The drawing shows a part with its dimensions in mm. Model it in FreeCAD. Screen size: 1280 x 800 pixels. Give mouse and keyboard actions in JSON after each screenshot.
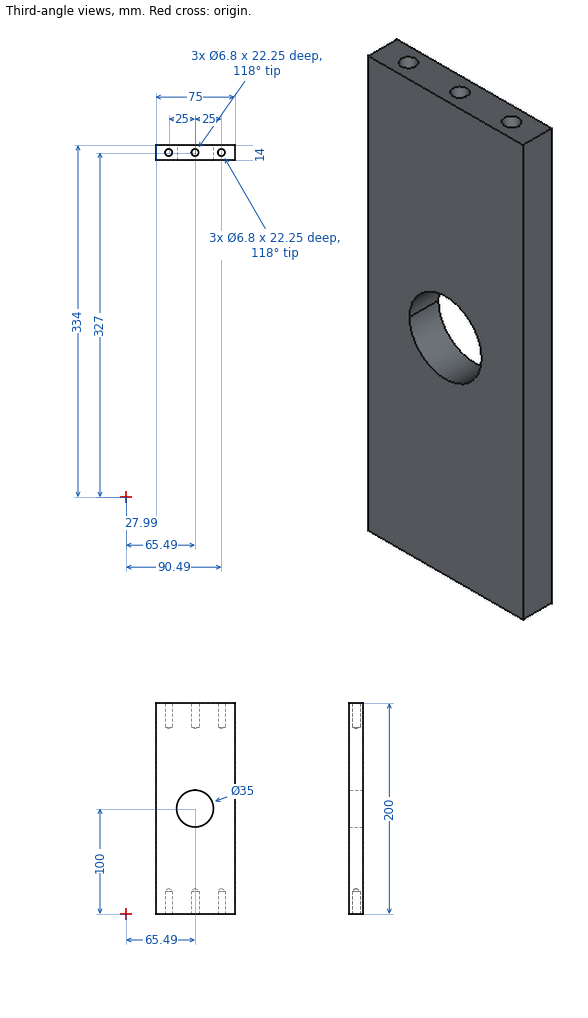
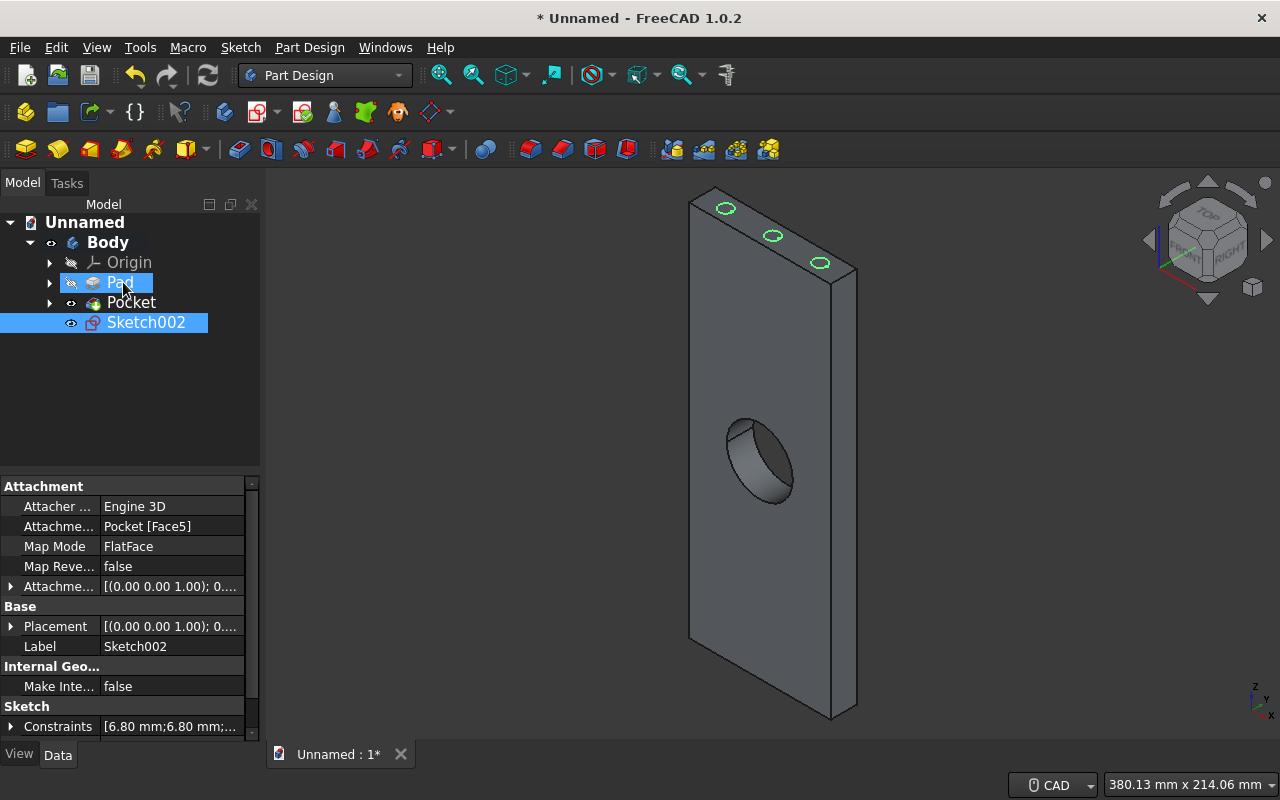
{"action": "left_click", "coordinate": [272, 150]}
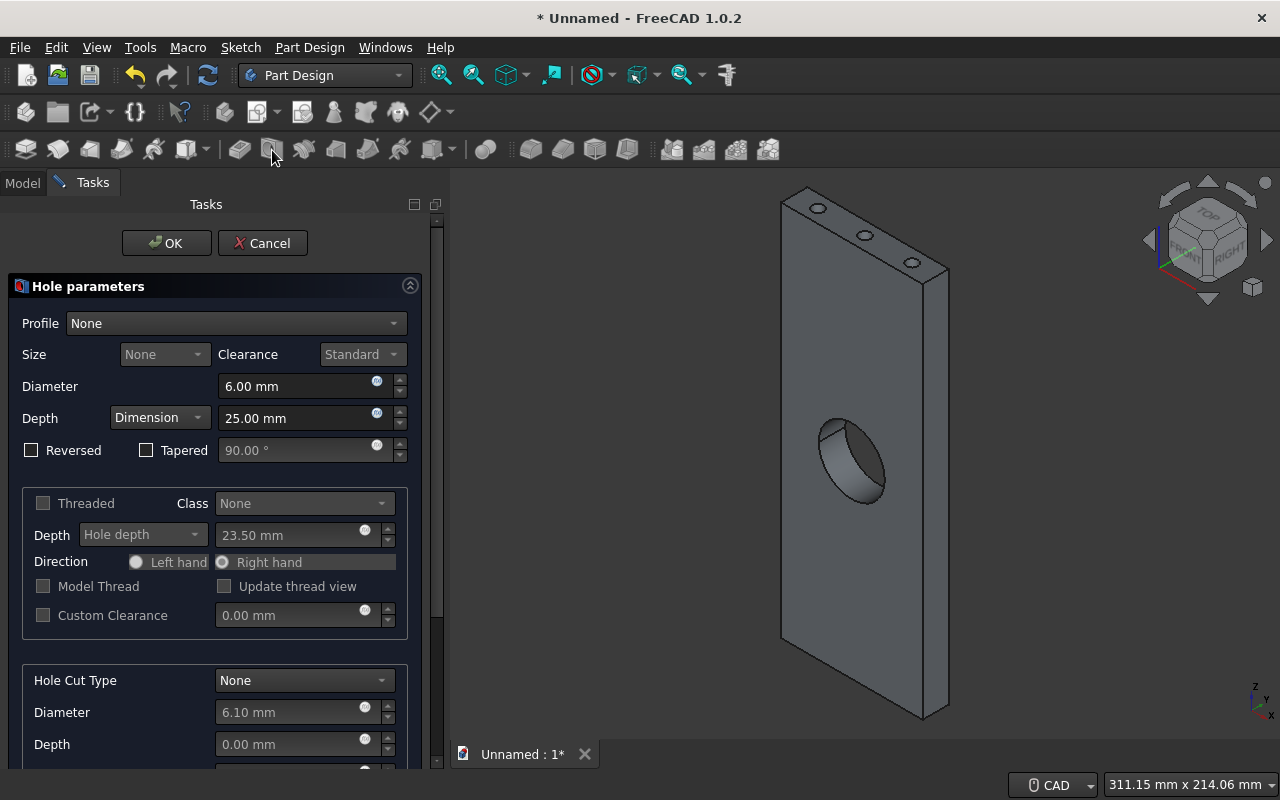
{"action": "triple_click", "coordinate": [305, 386]}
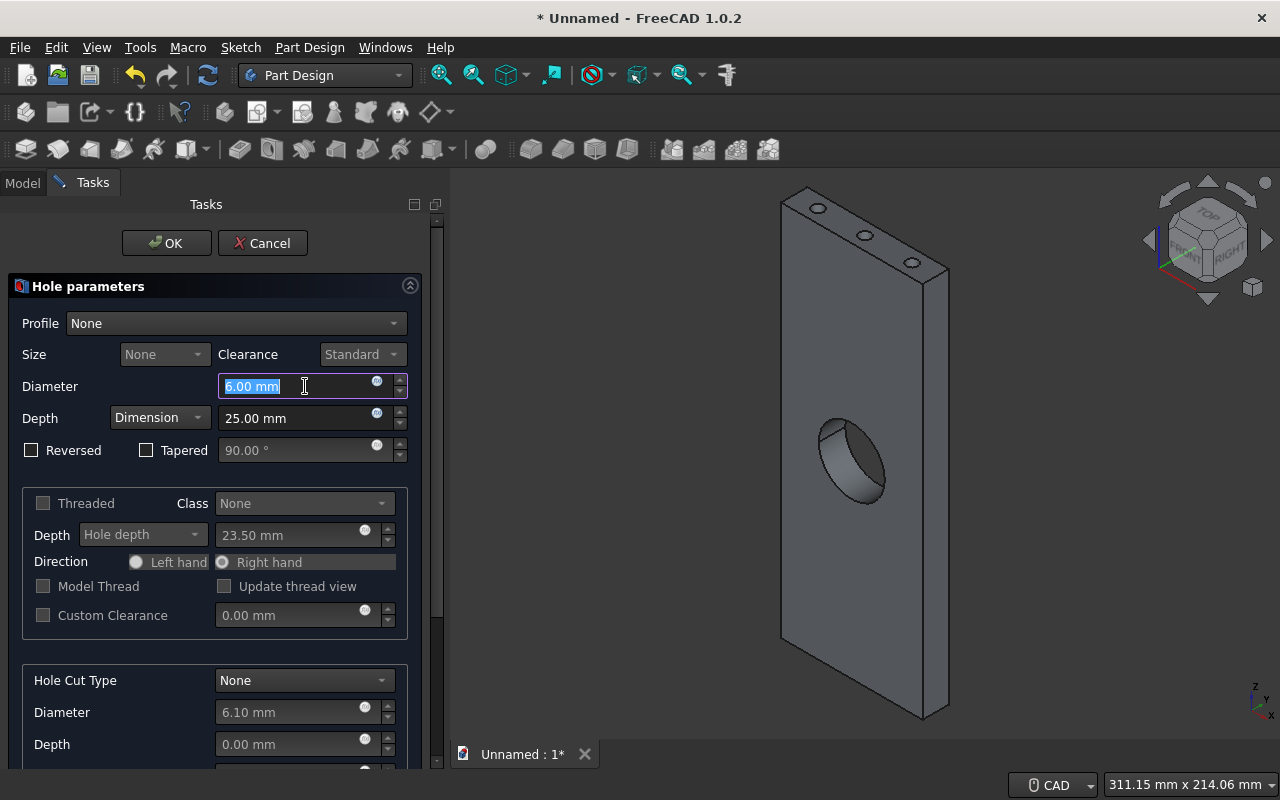
{"action": "type", "text": "6.8"}
{"action": "key", "text": "Tab"}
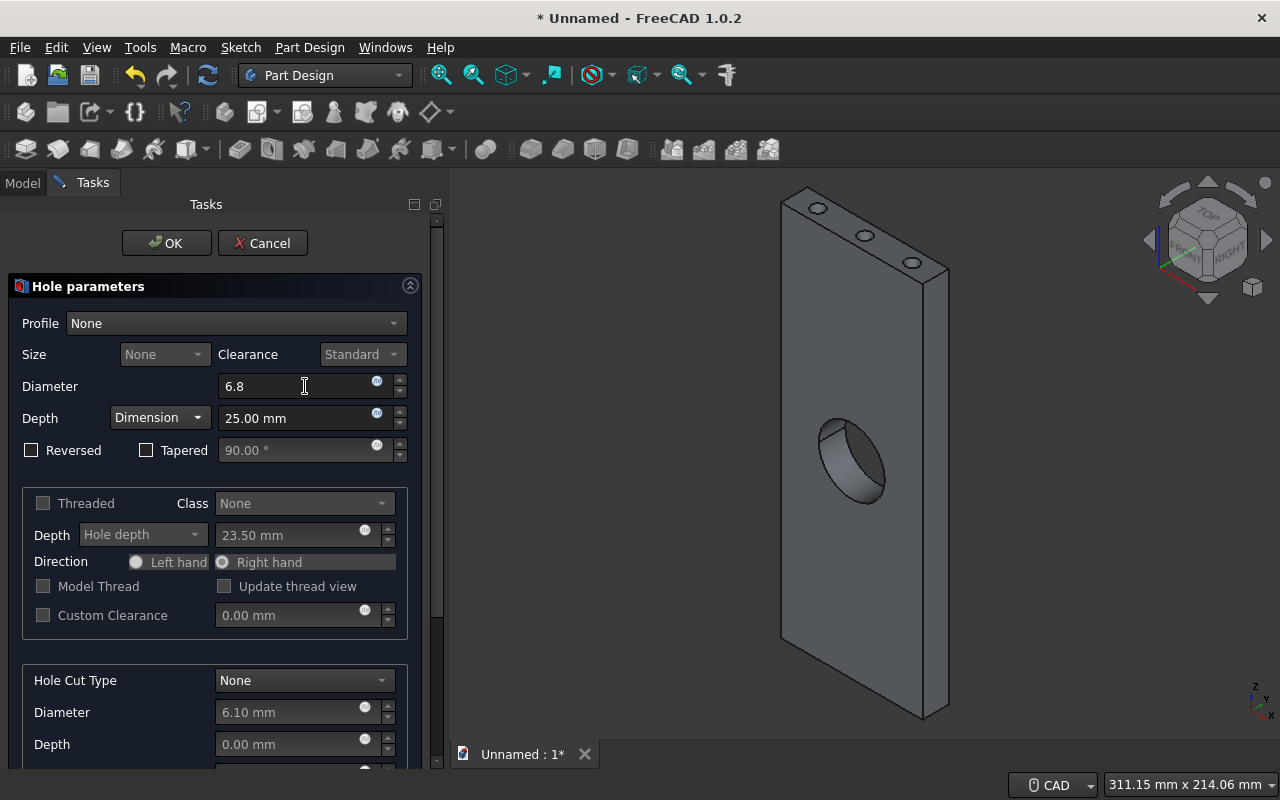
{"action": "triple_click", "coordinate": [305, 418]}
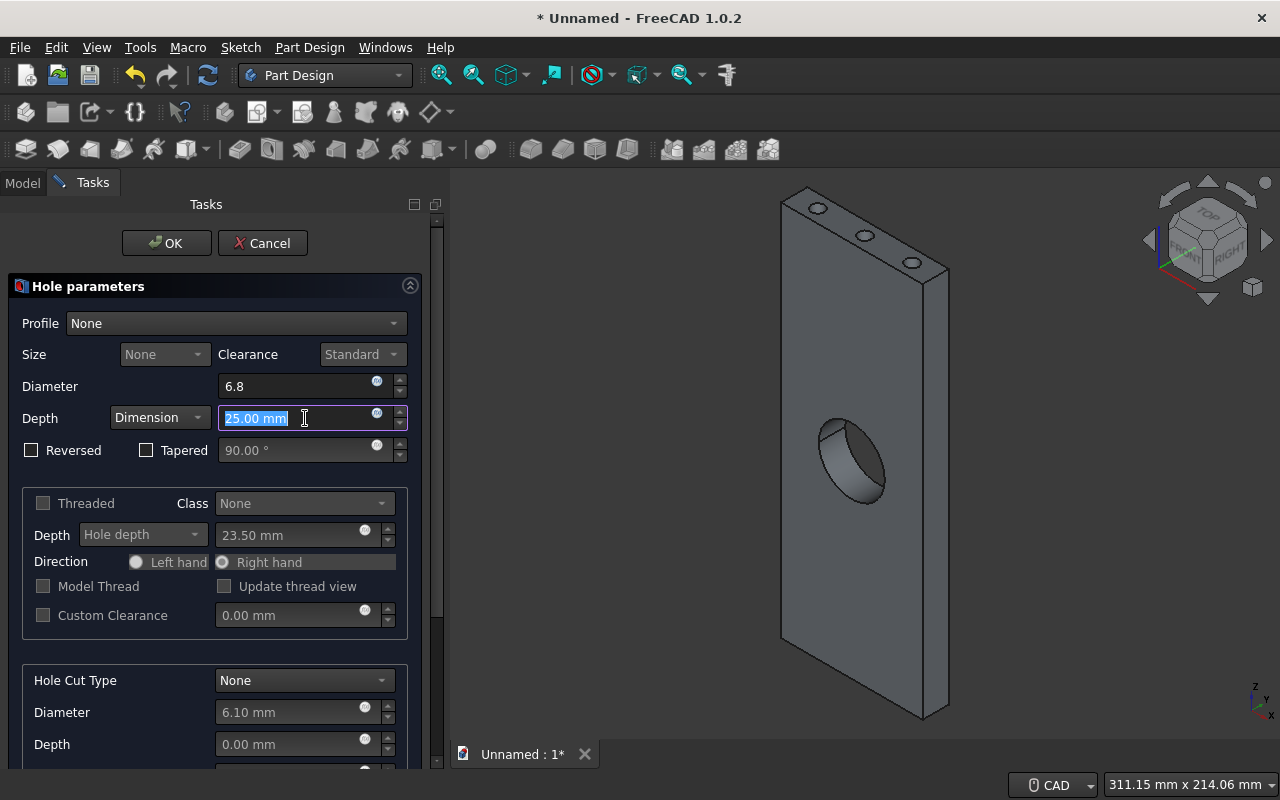
{"action": "type", "text": "22.25"}
{"action": "key", "text": "Tab"}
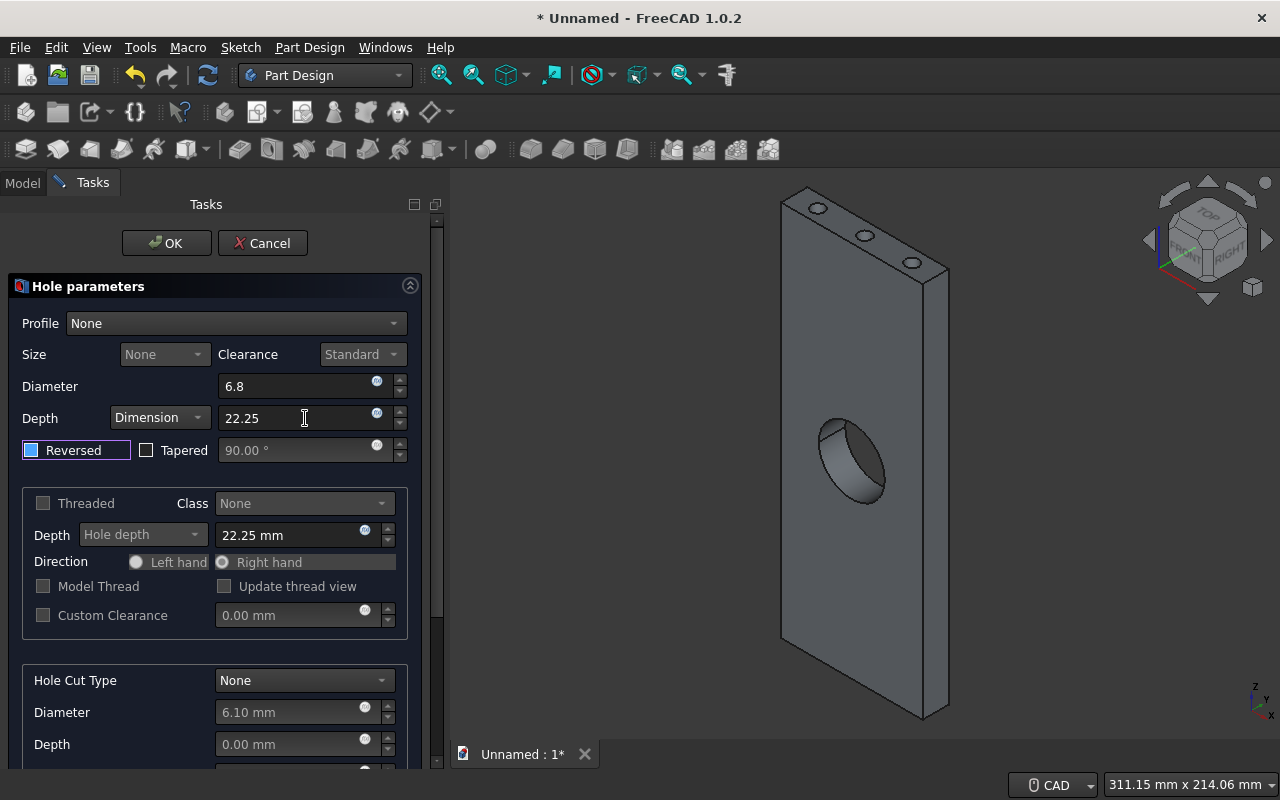
{"action": "left_click", "coordinate": [167, 243]}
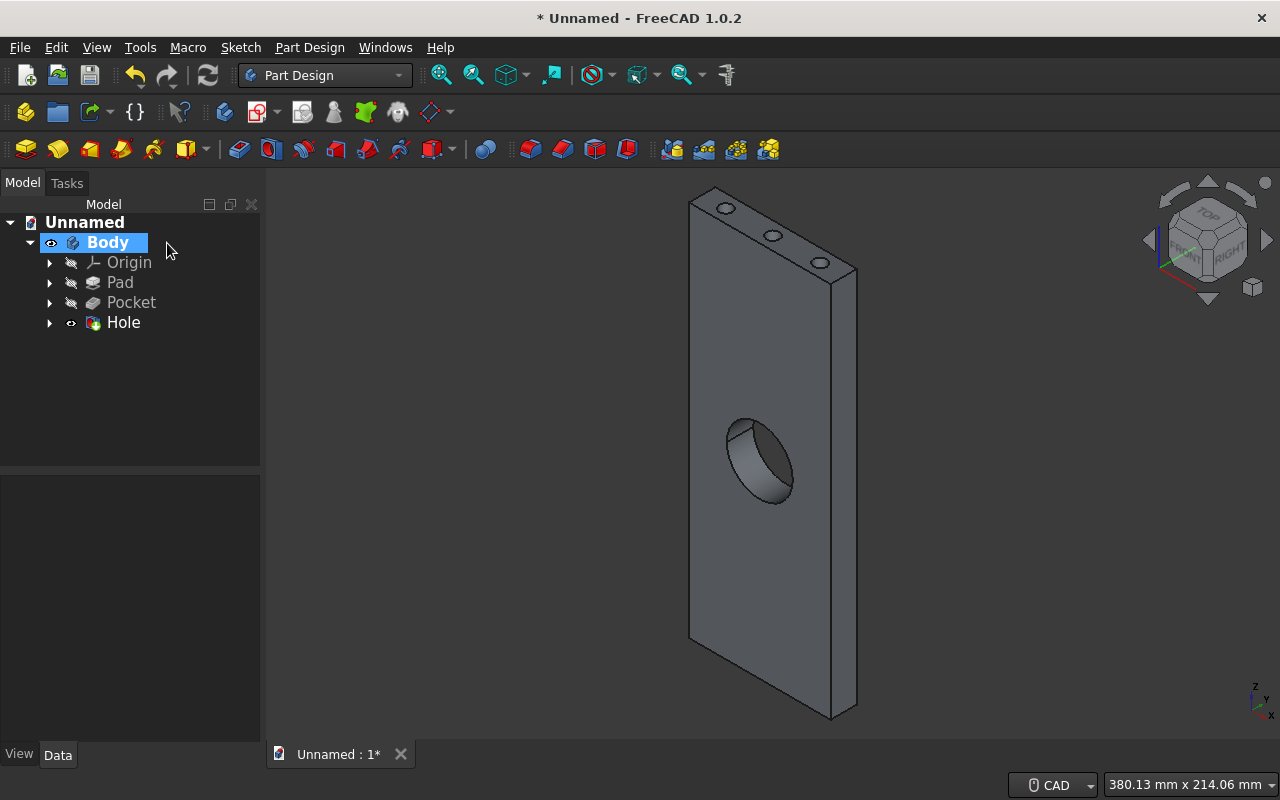
{"action": "left_click", "coordinate": [258, 112]}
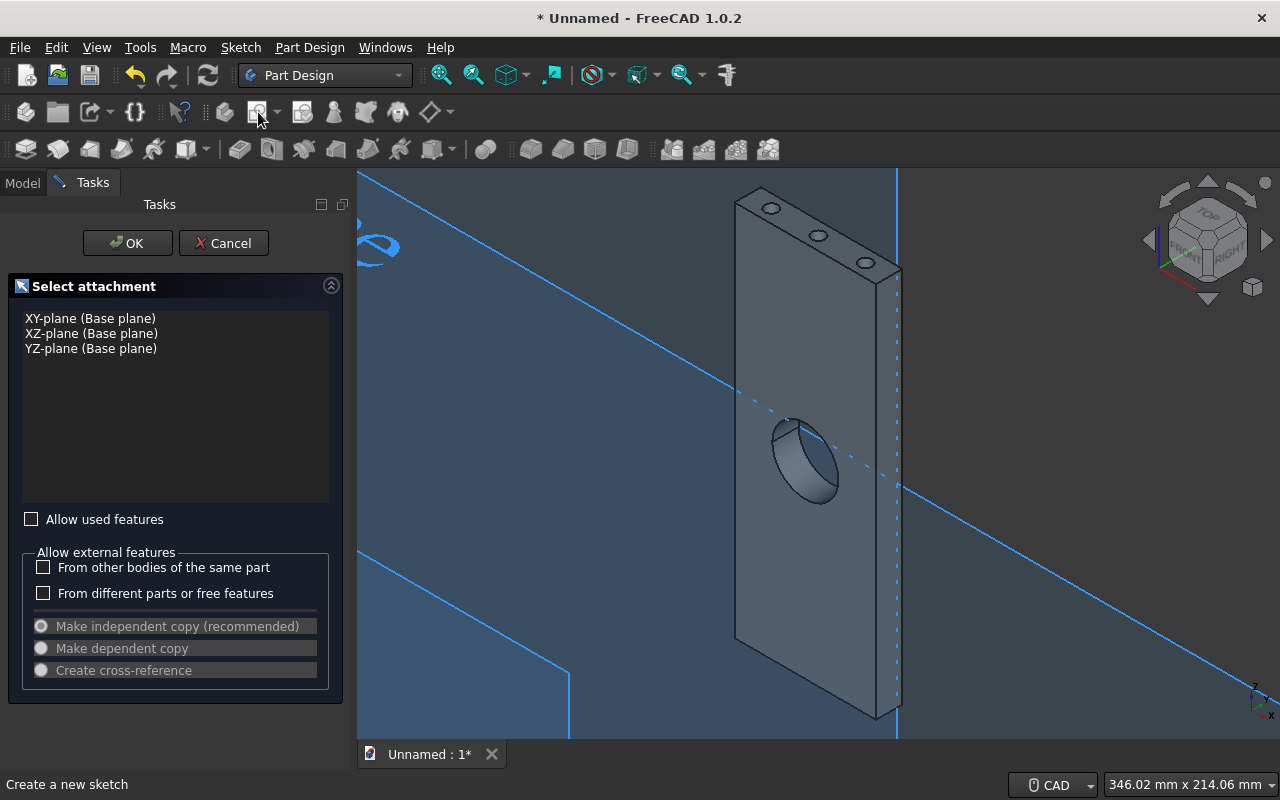
{"action": "left_click", "coordinate": [82, 318]}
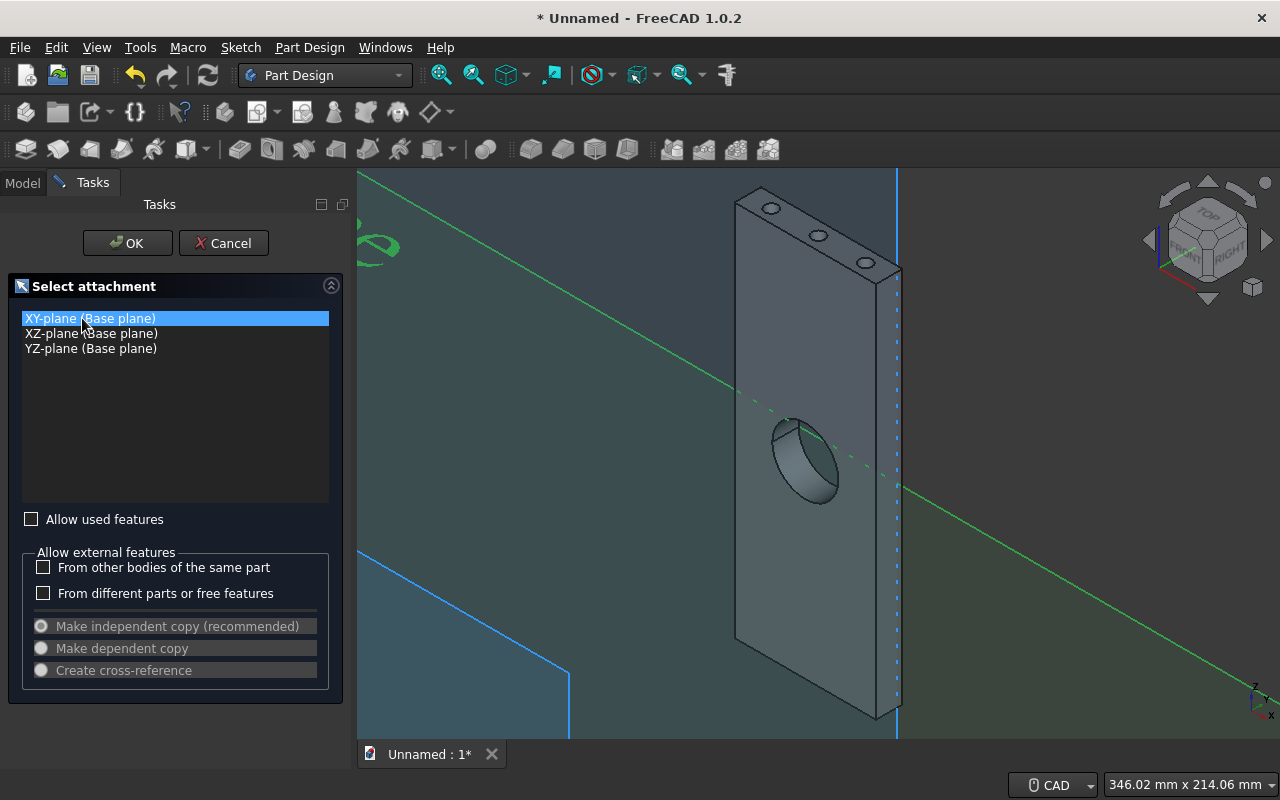
{"action": "left_click", "coordinate": [128, 243]}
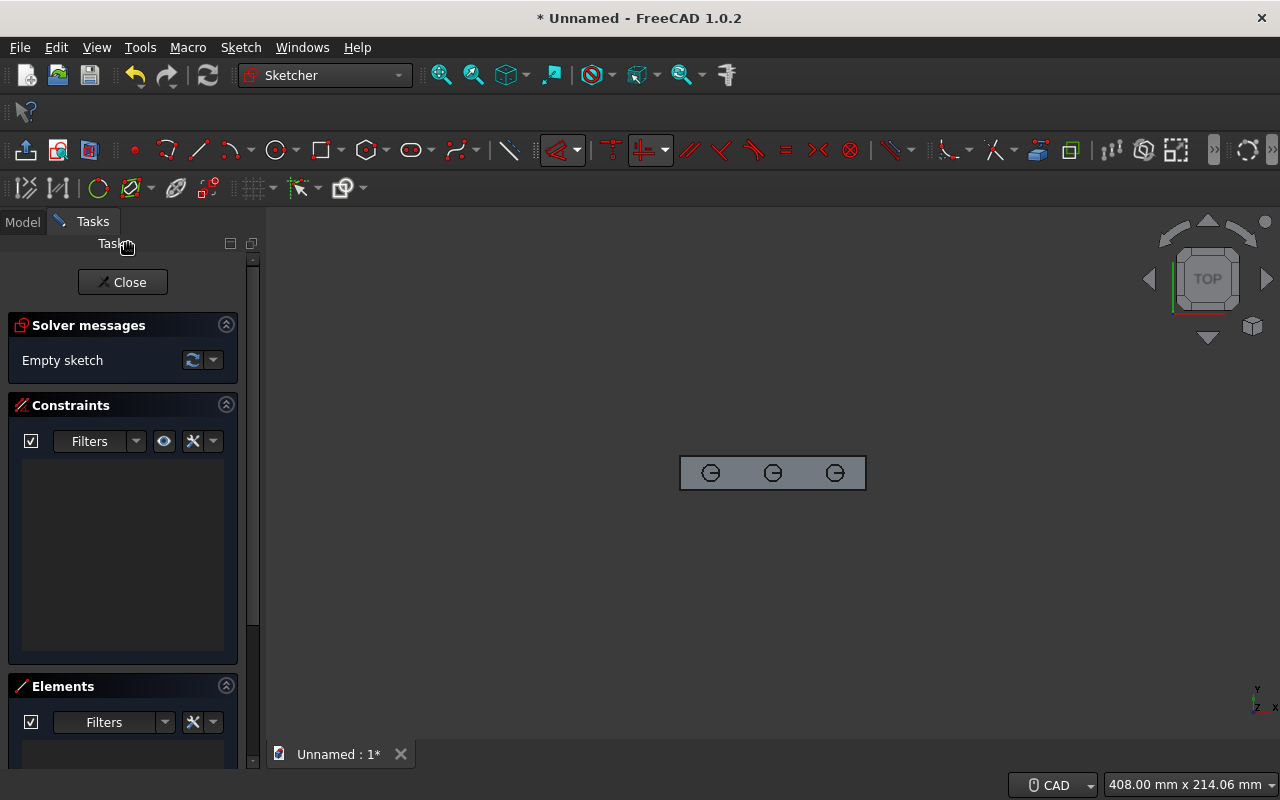
{"action": "left_click", "coordinate": [90, 150]}